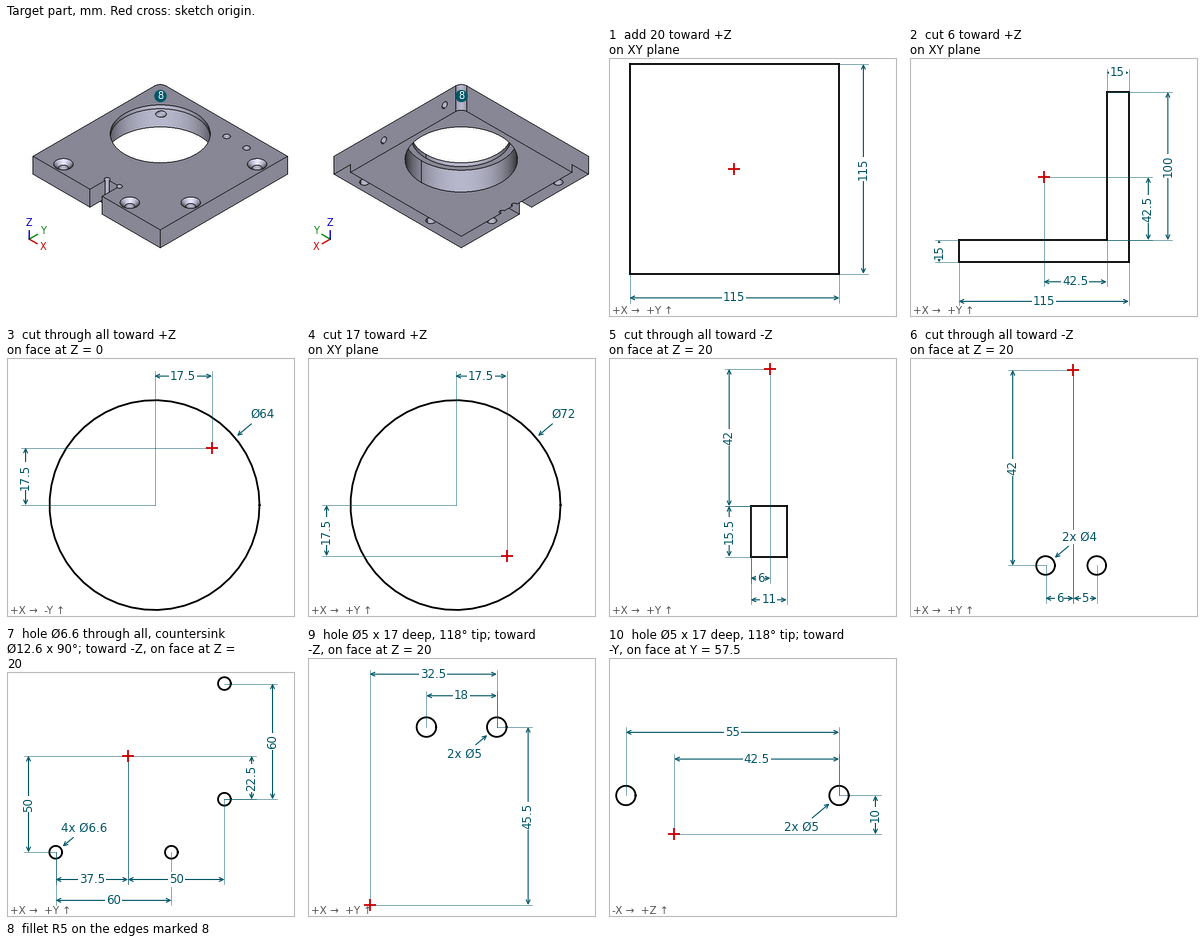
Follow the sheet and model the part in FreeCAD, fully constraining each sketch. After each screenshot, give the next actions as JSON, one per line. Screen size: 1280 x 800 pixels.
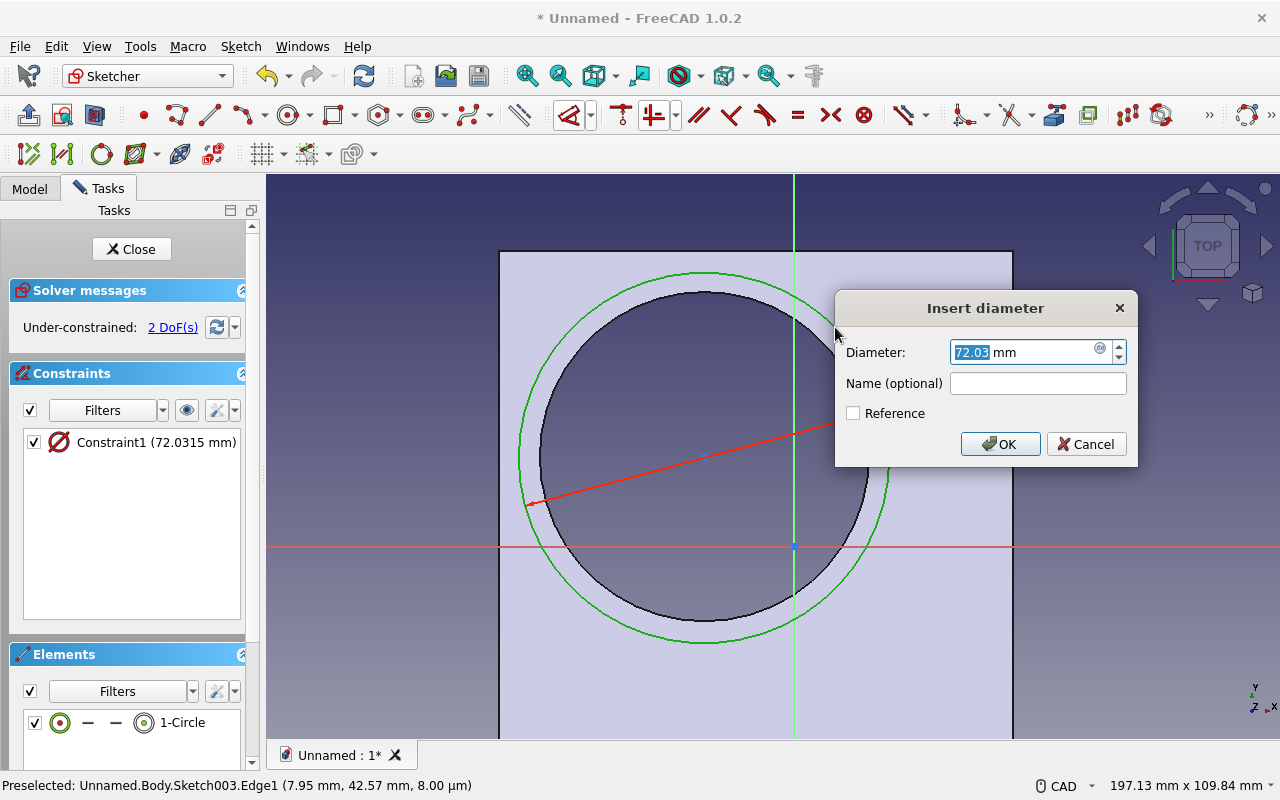
{"action": "type", "text": "72"}
{"action": "key", "text": "Return"}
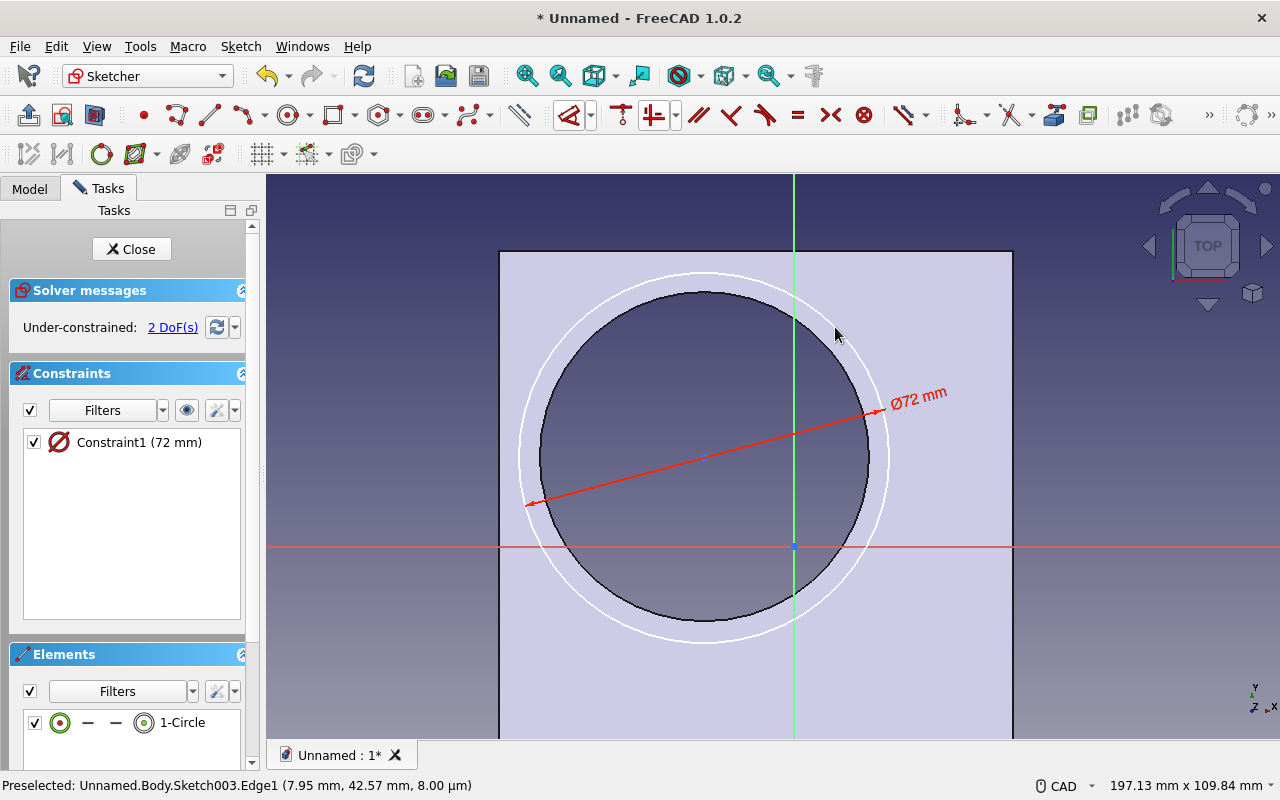
{"action": "left_click", "coordinate": [704, 458]}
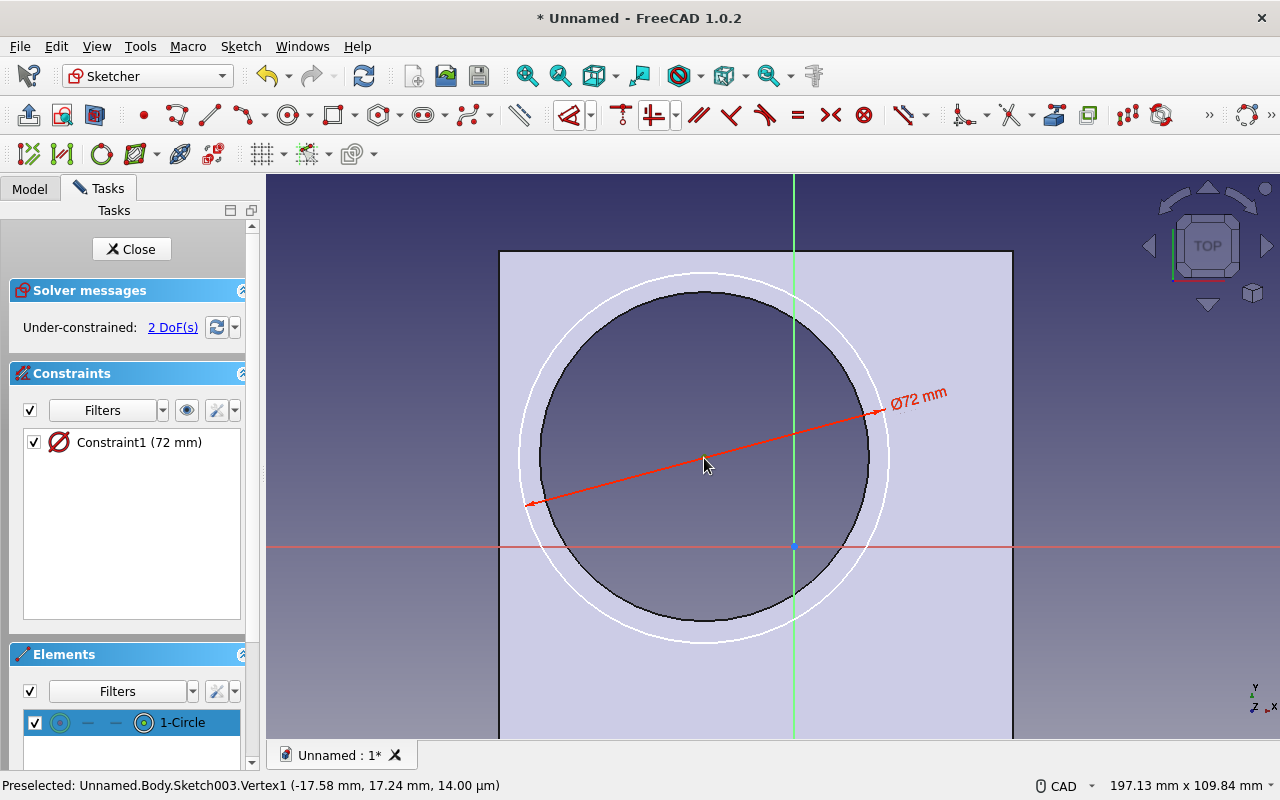
{"action": "key", "text": "l"}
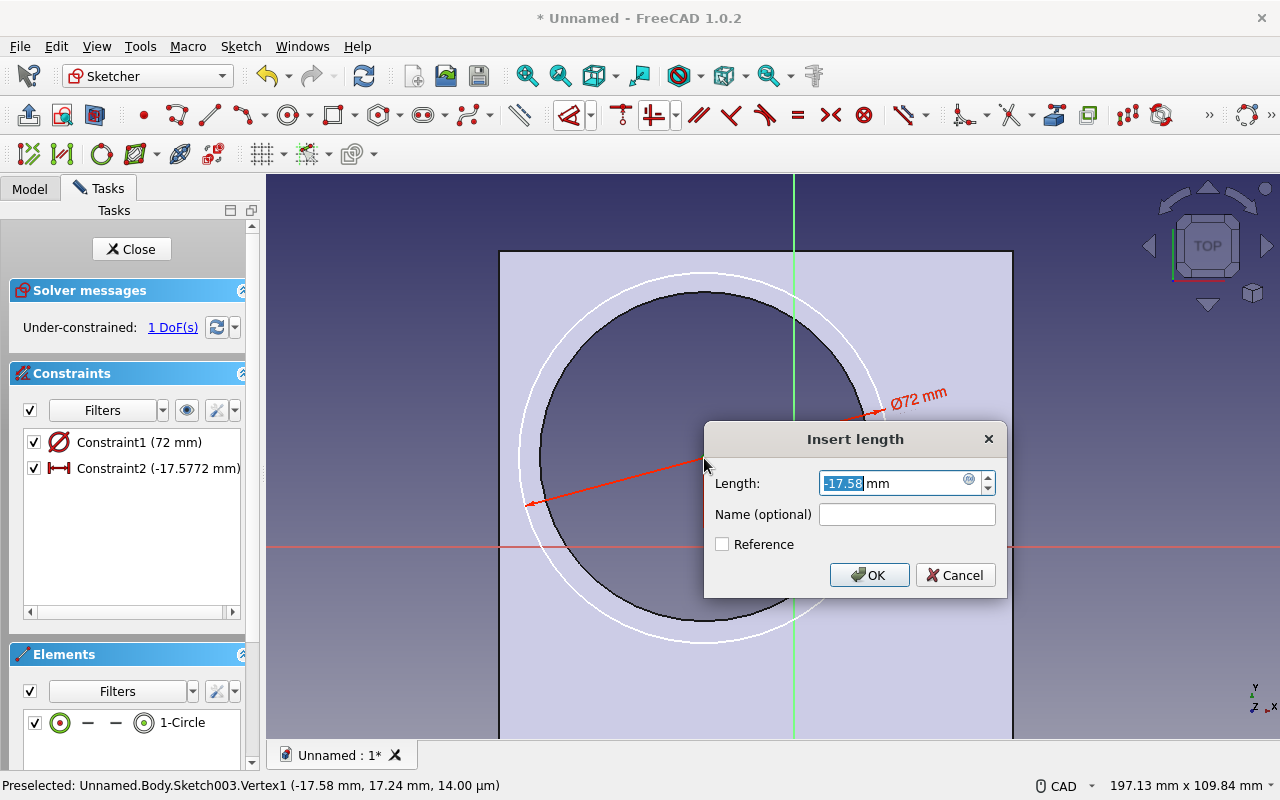
{"action": "type", "text": "-17.5"}
{"action": "key", "text": "Return"}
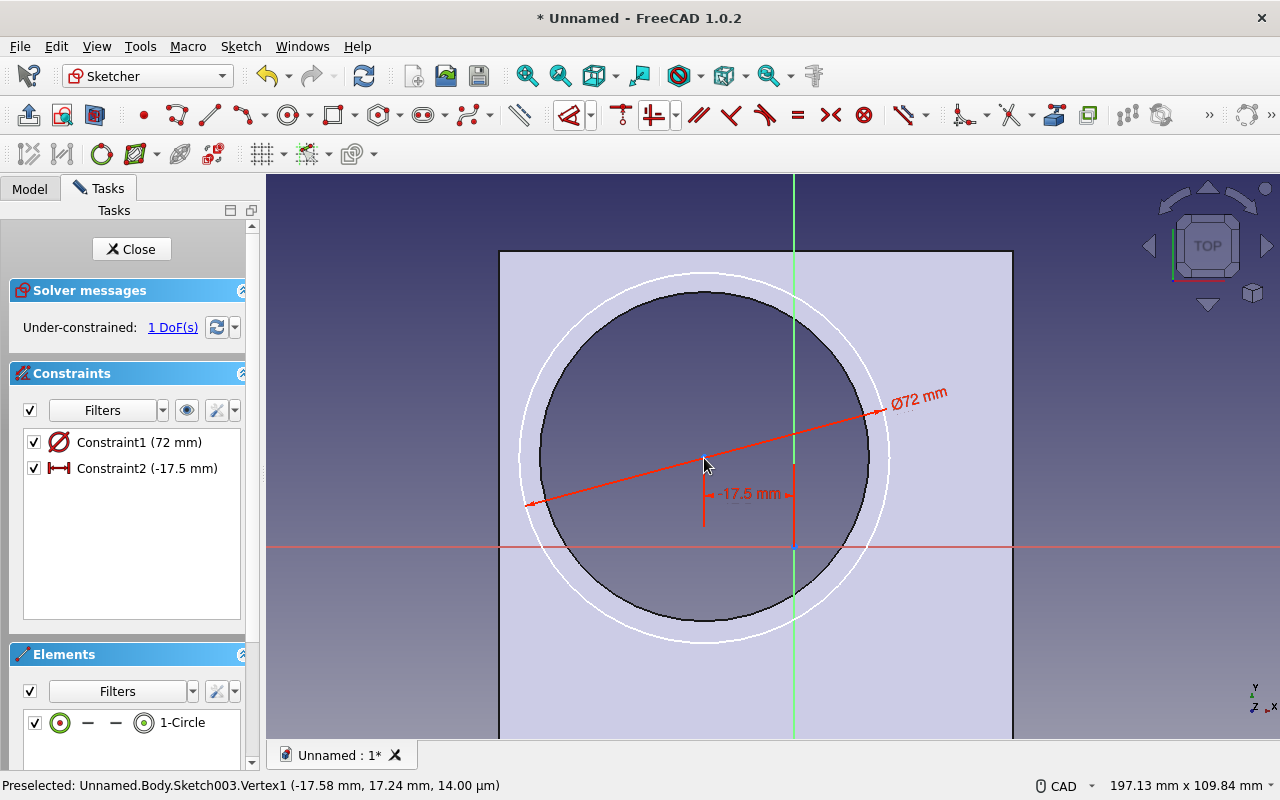
{"action": "left_click", "coordinate": [704, 458]}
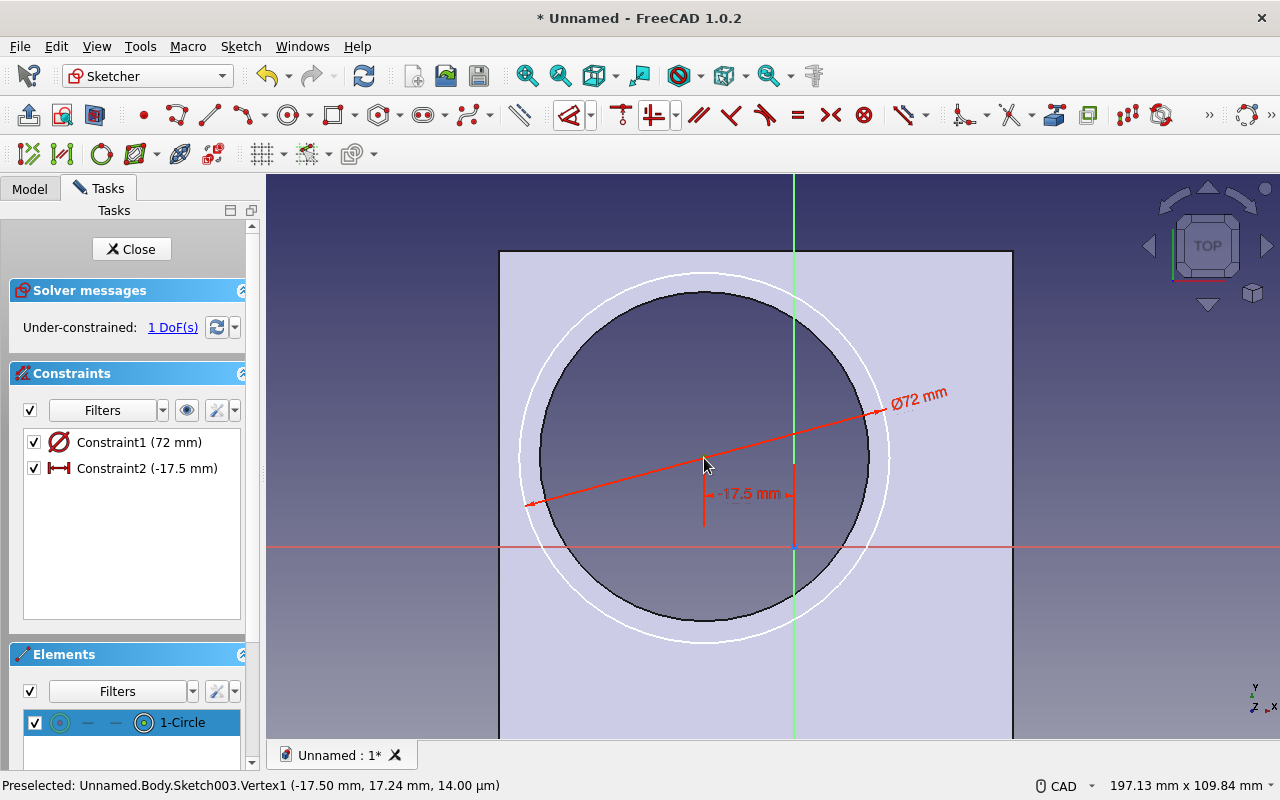
{"action": "left_click", "coordinate": [590, 116]}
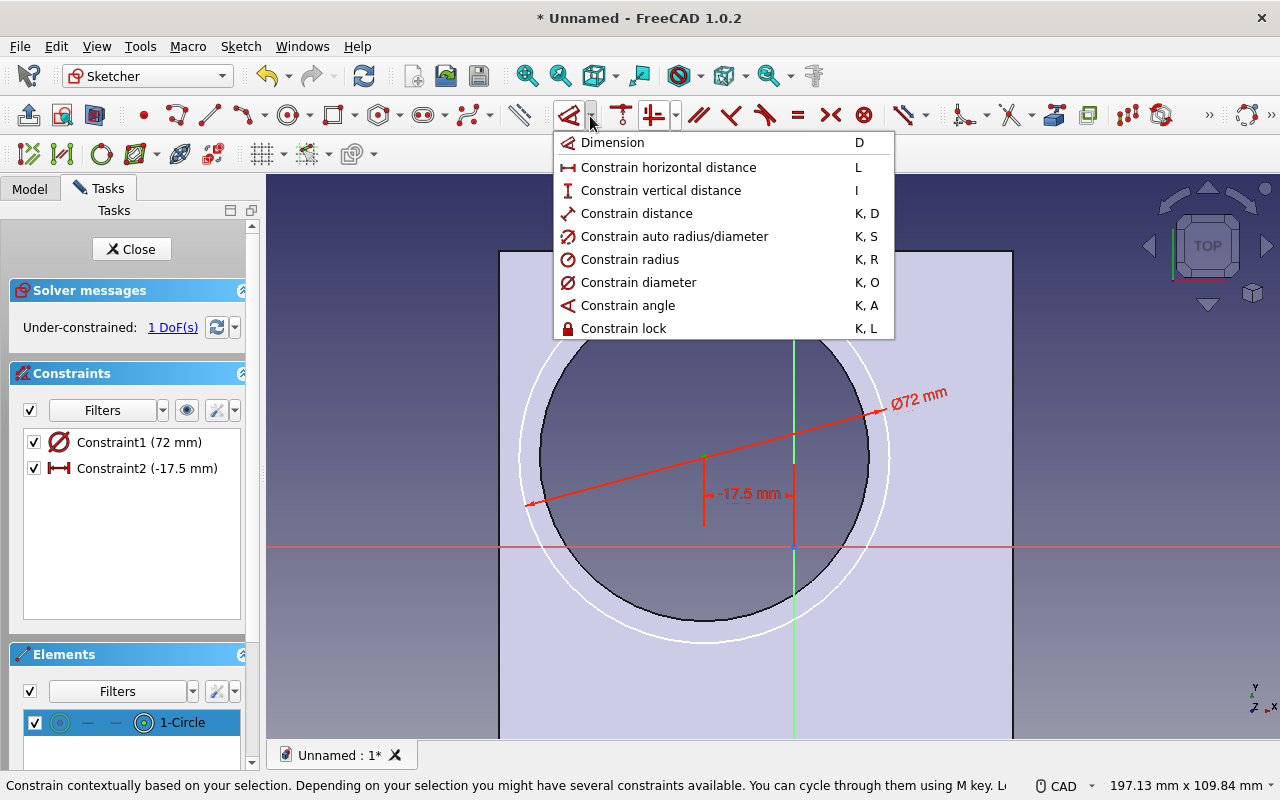
{"action": "left_click", "coordinate": [724, 190]}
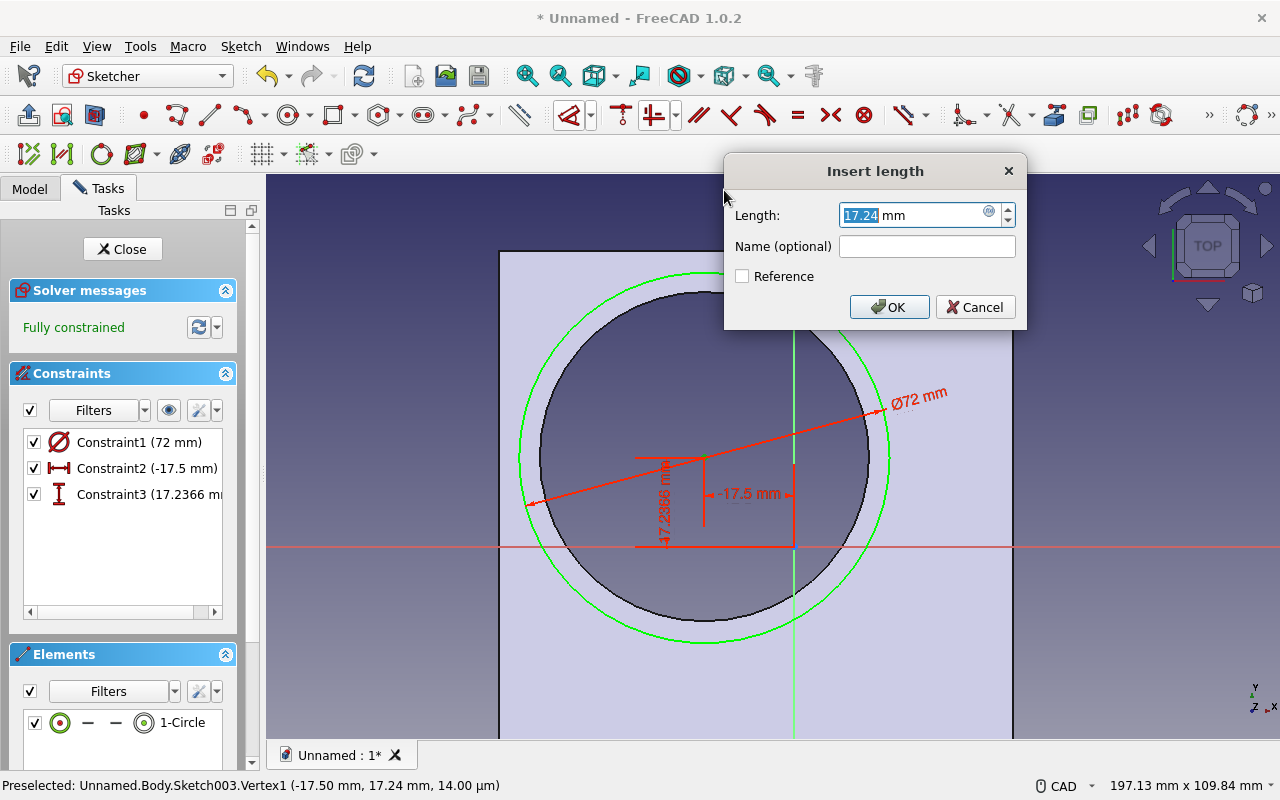
{"action": "type", "text": "17.5"}
{"action": "key", "text": "Return"}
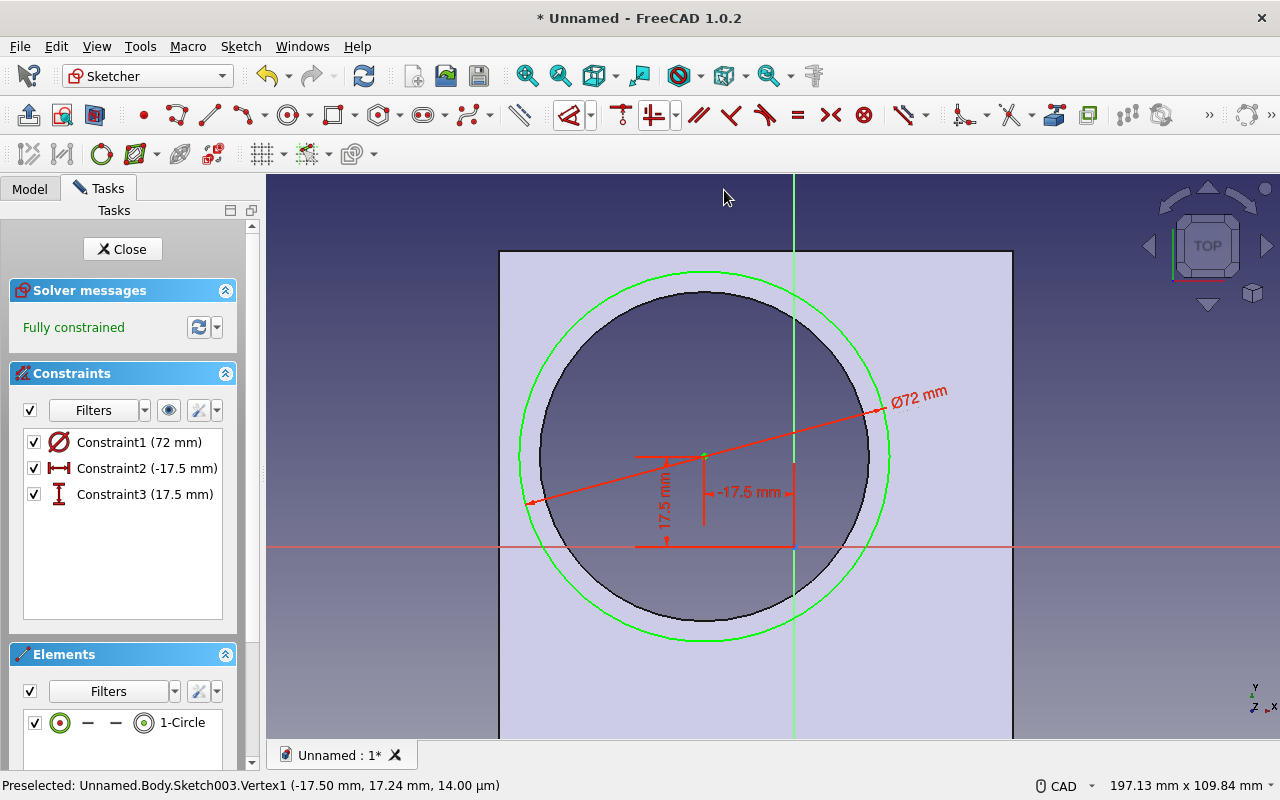
{"action": "left_click", "coordinate": [123, 249]}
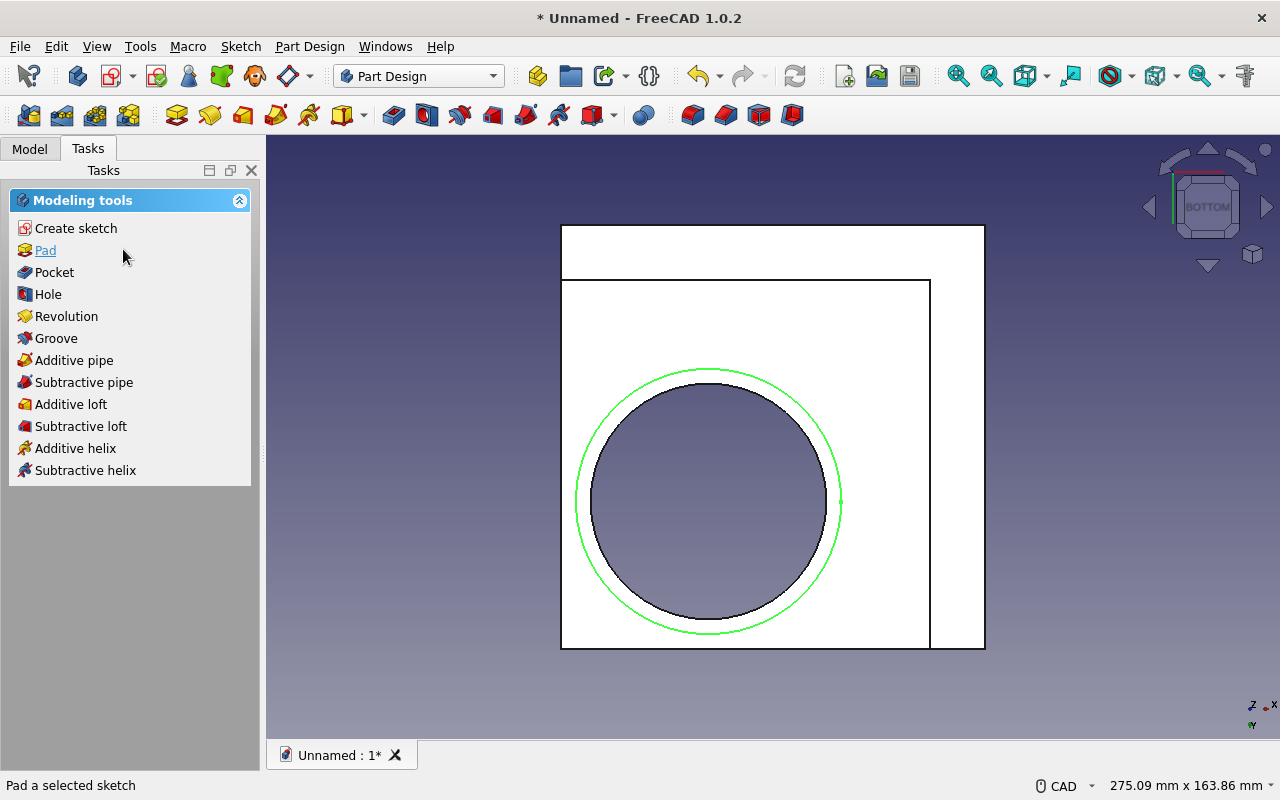
{"action": "left_click", "coordinate": [394, 116]}